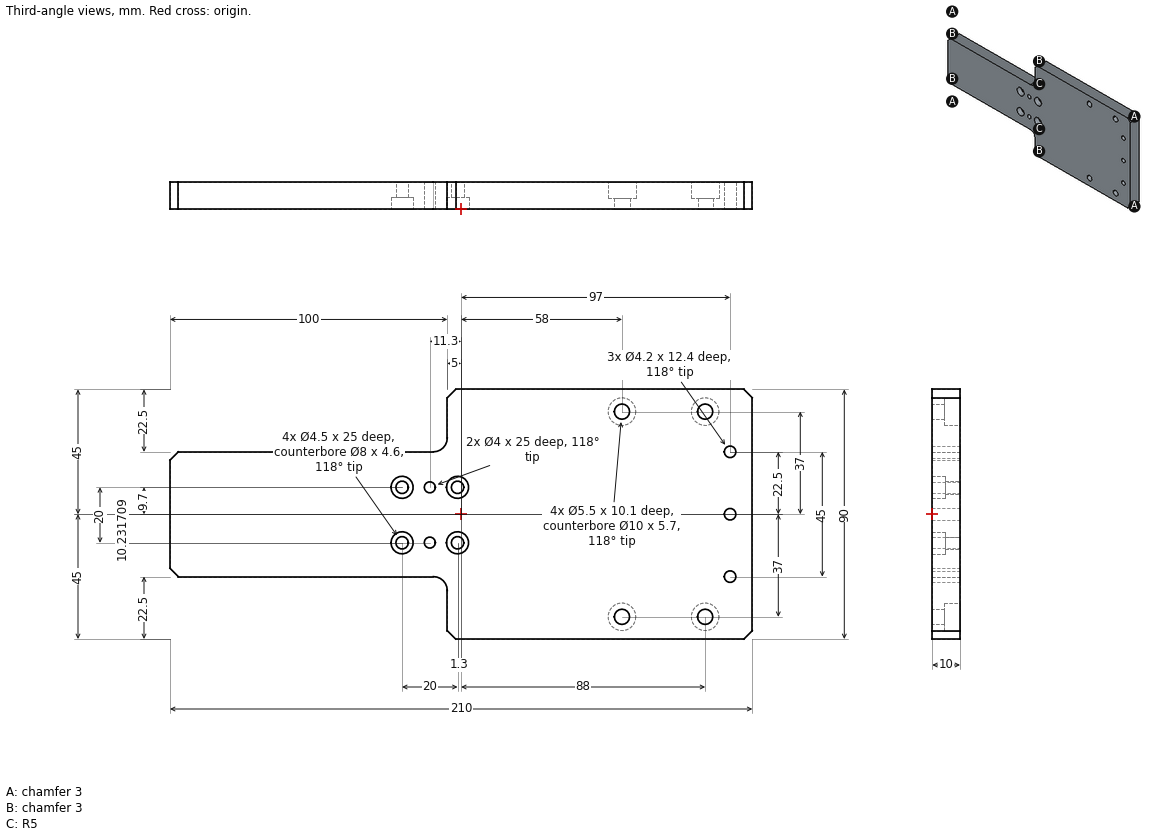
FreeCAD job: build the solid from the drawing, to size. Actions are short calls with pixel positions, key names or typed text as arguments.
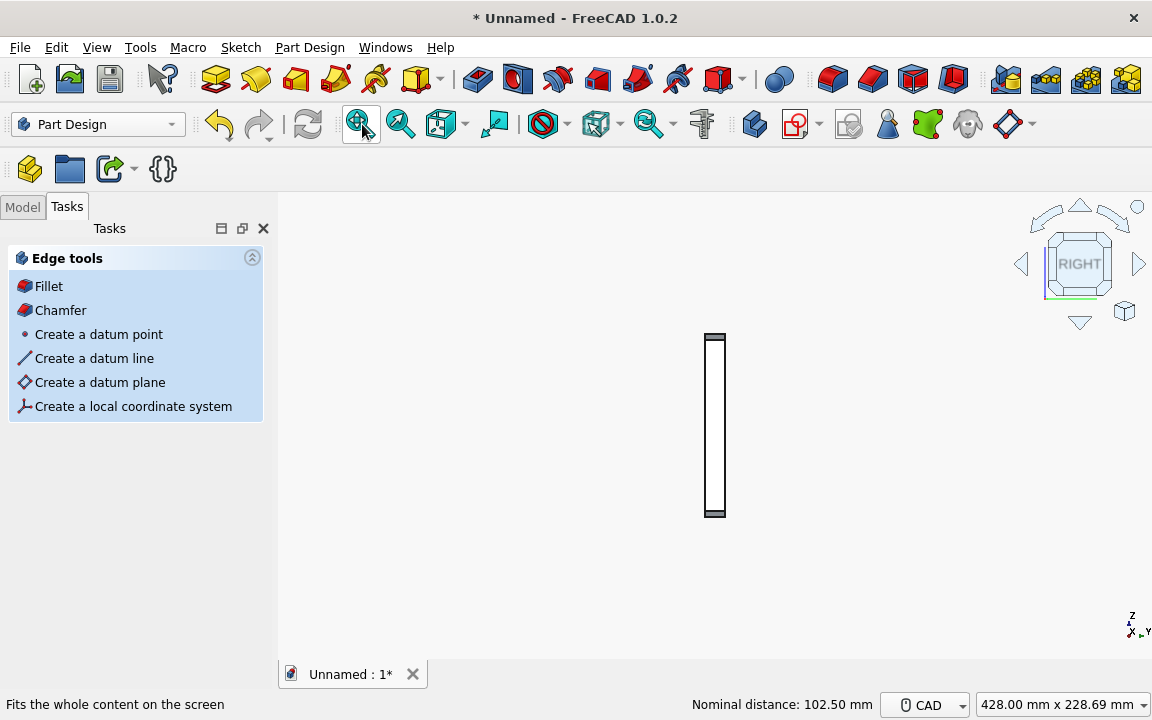
key(5)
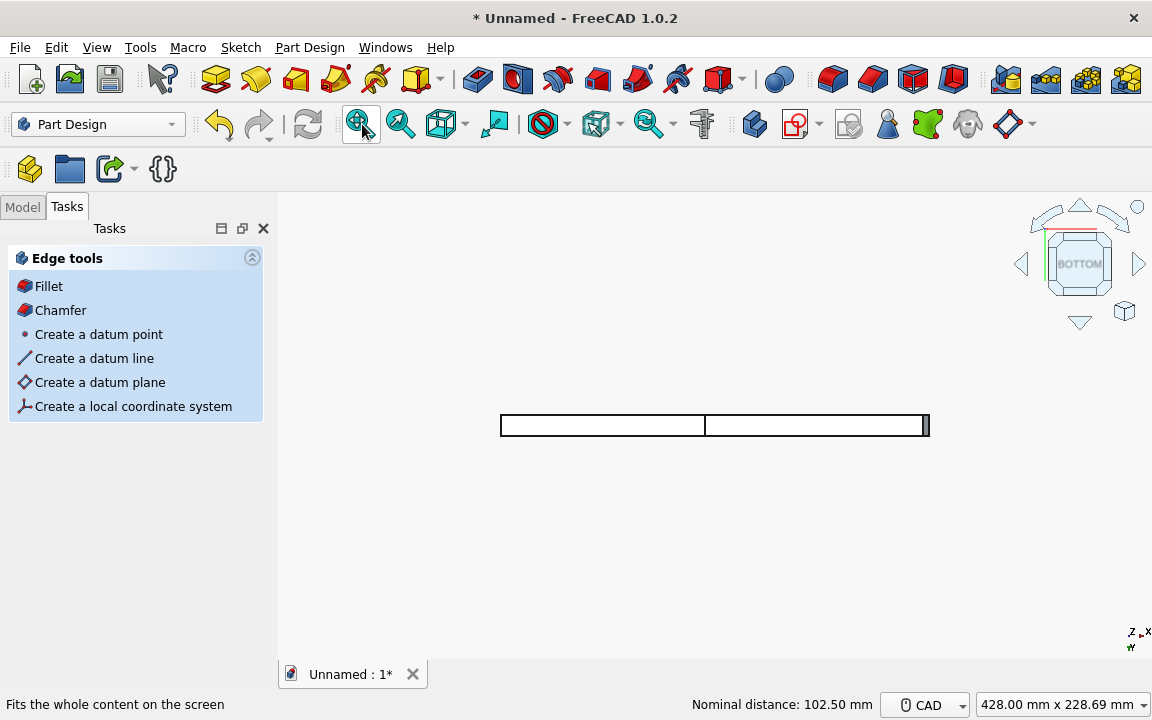
click(705, 424, ctrl)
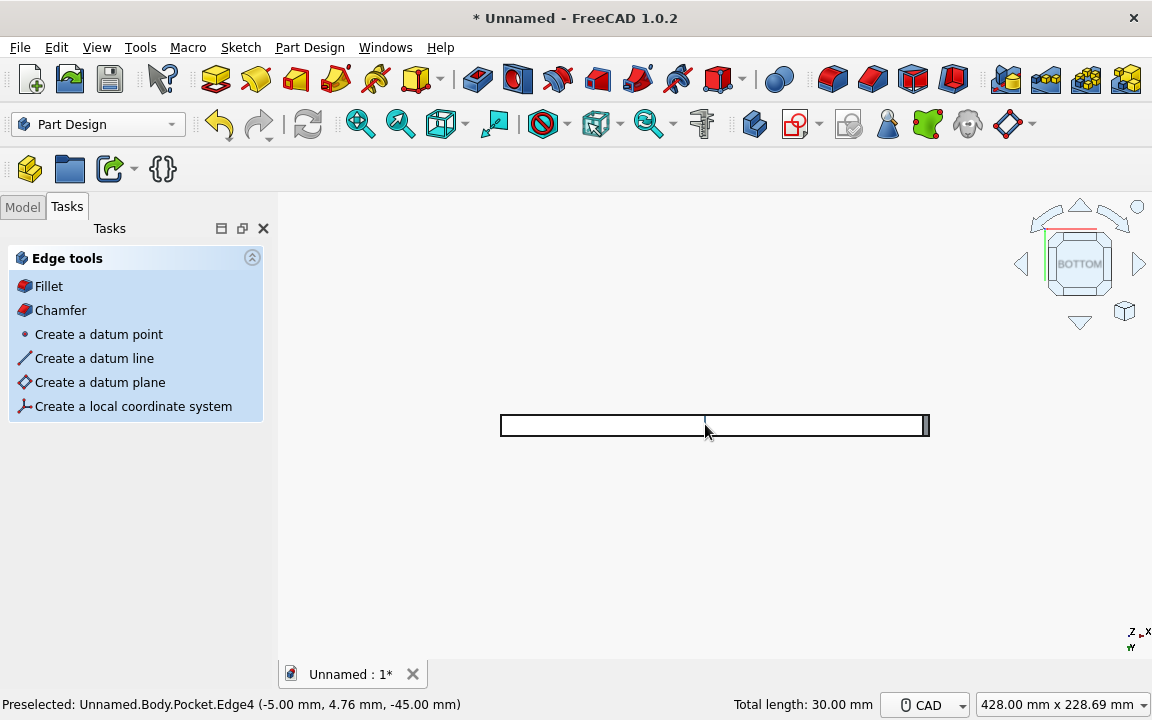
click(501, 424, ctrl)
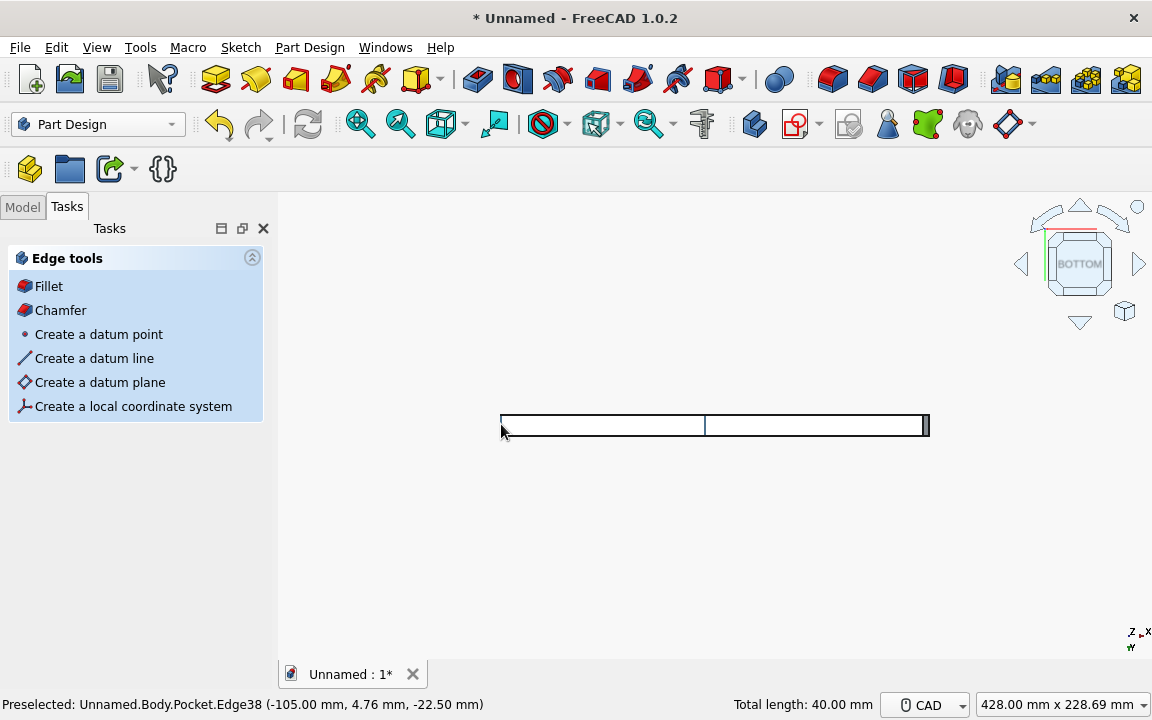
click(874, 80)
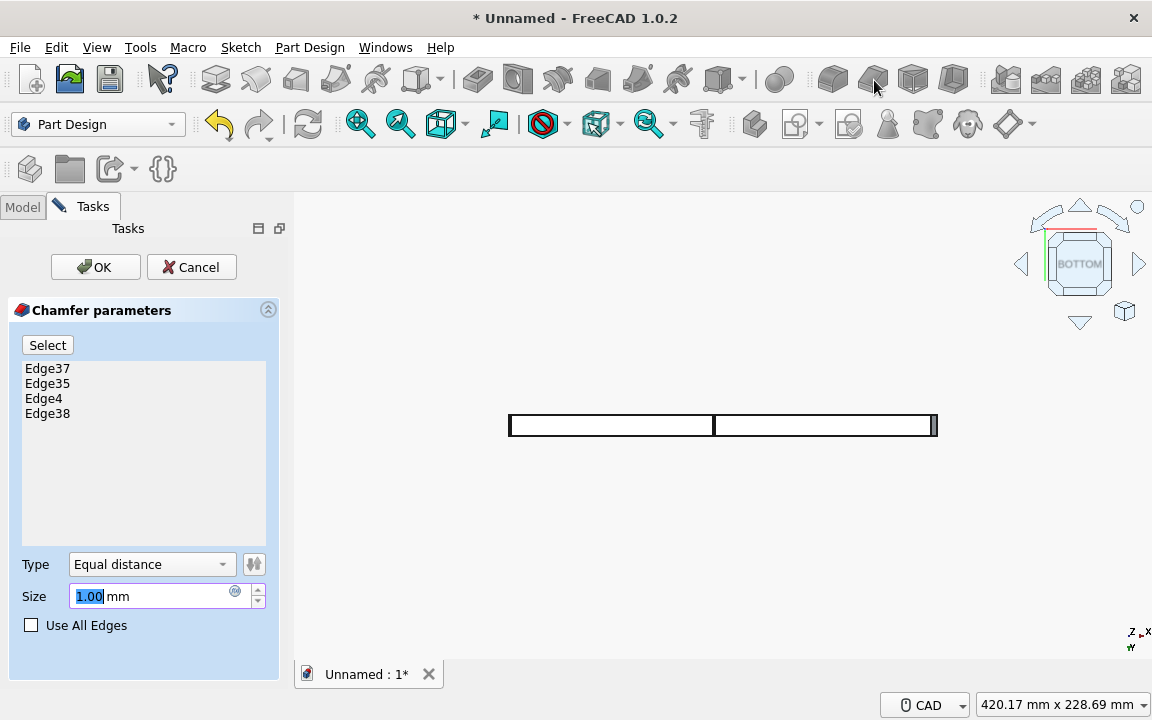
text(3)
key(Tab)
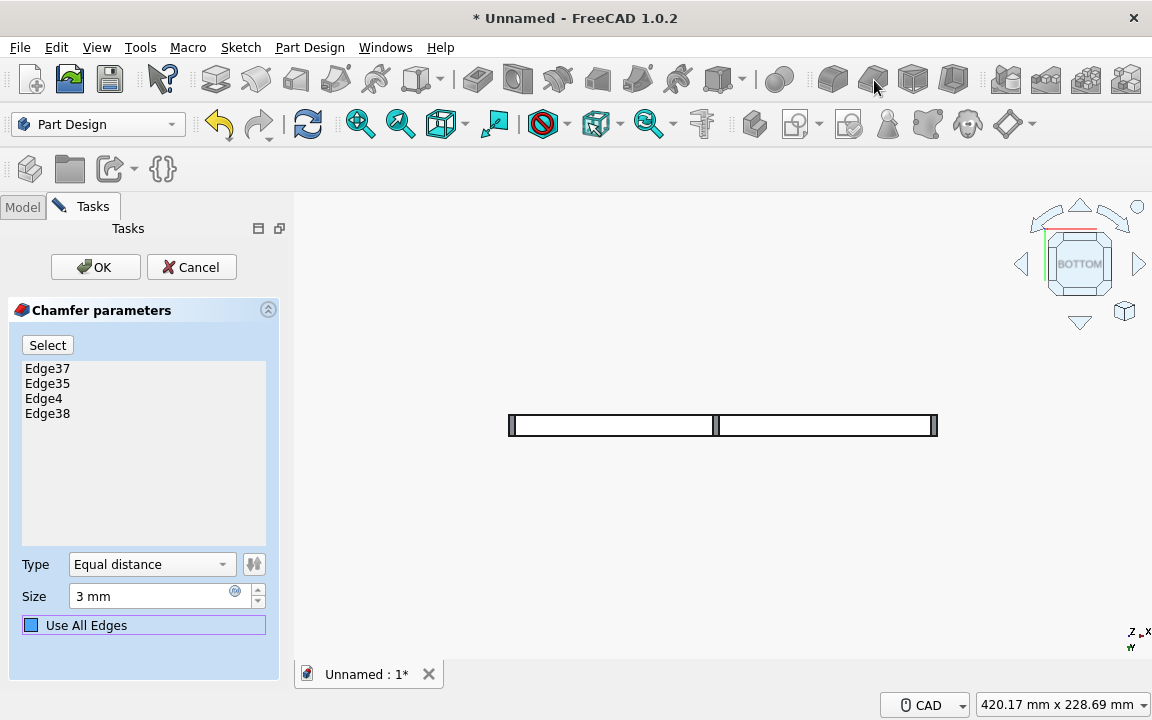
click(96, 267)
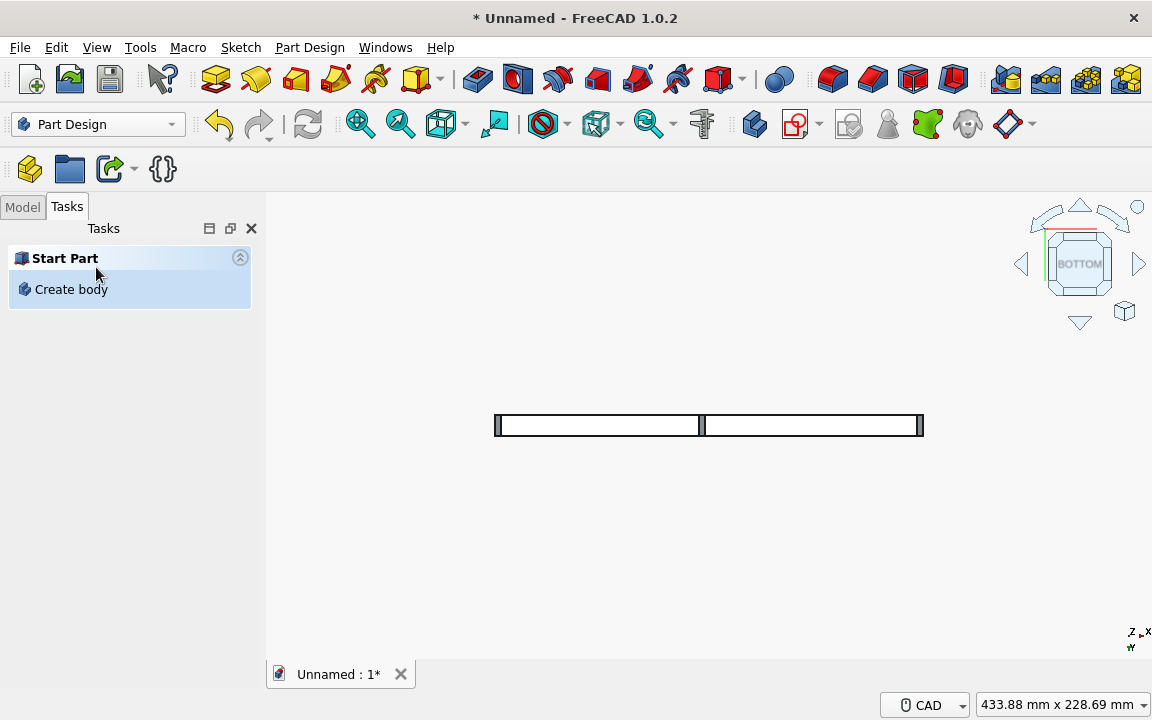
scroll(699, 424, up, 4)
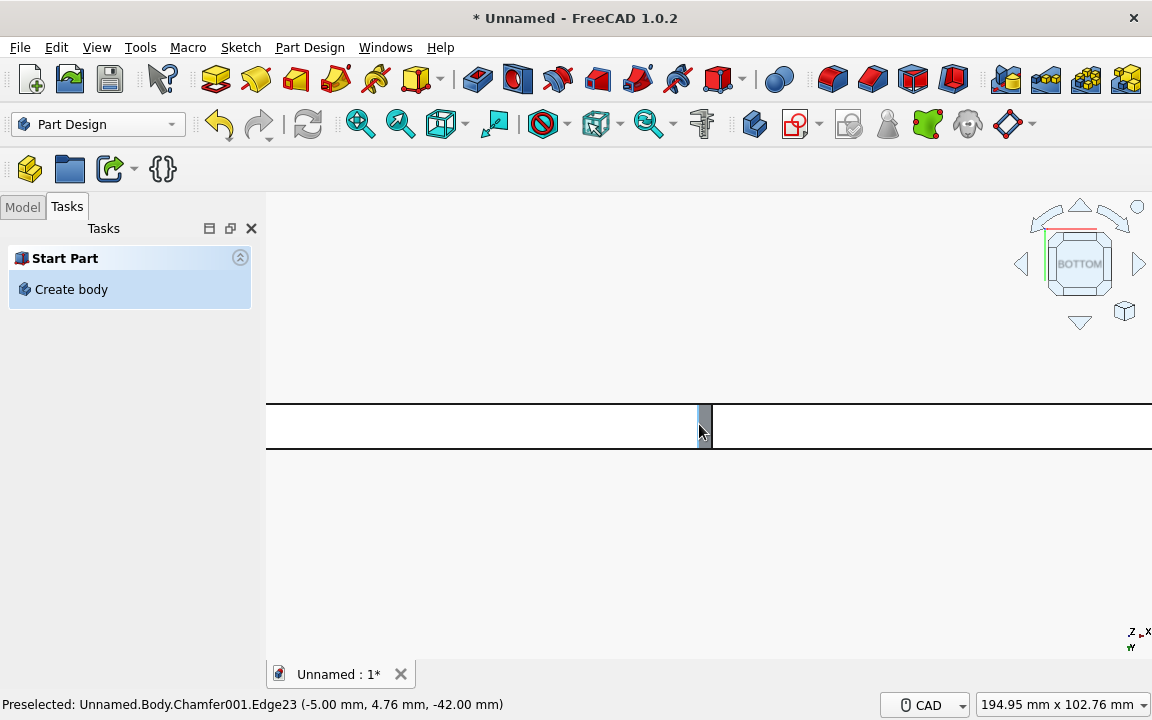
click(362, 124)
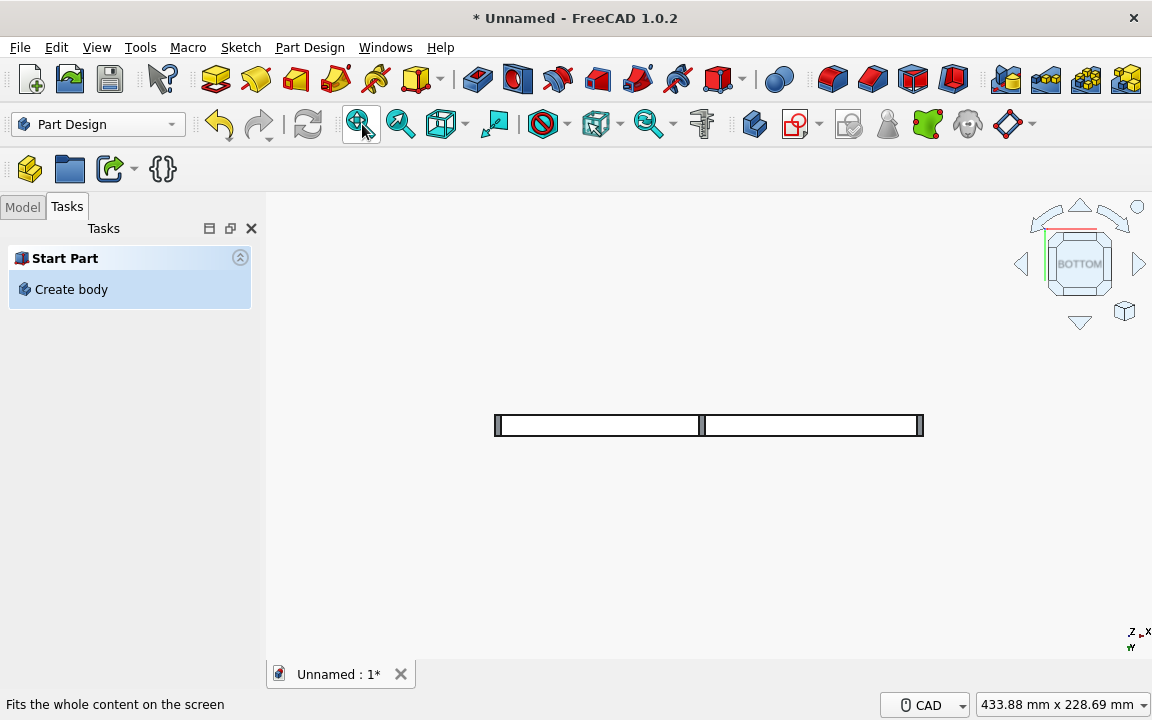
key(0)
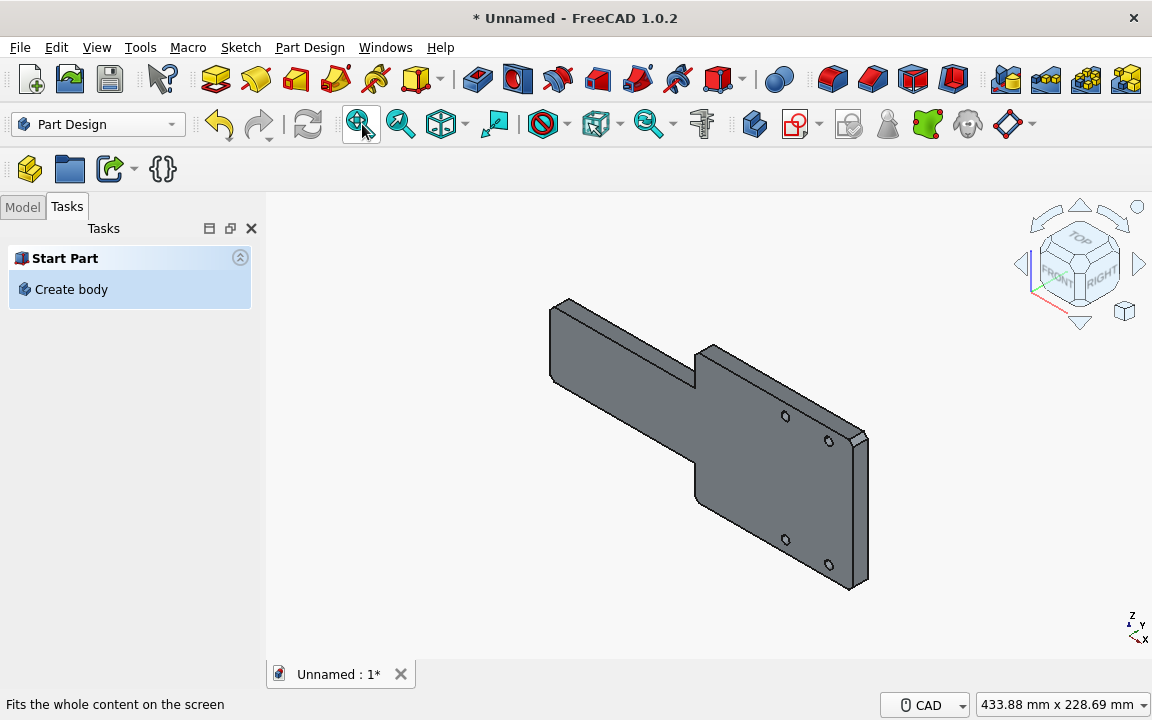
scroll(702, 383, up, 4)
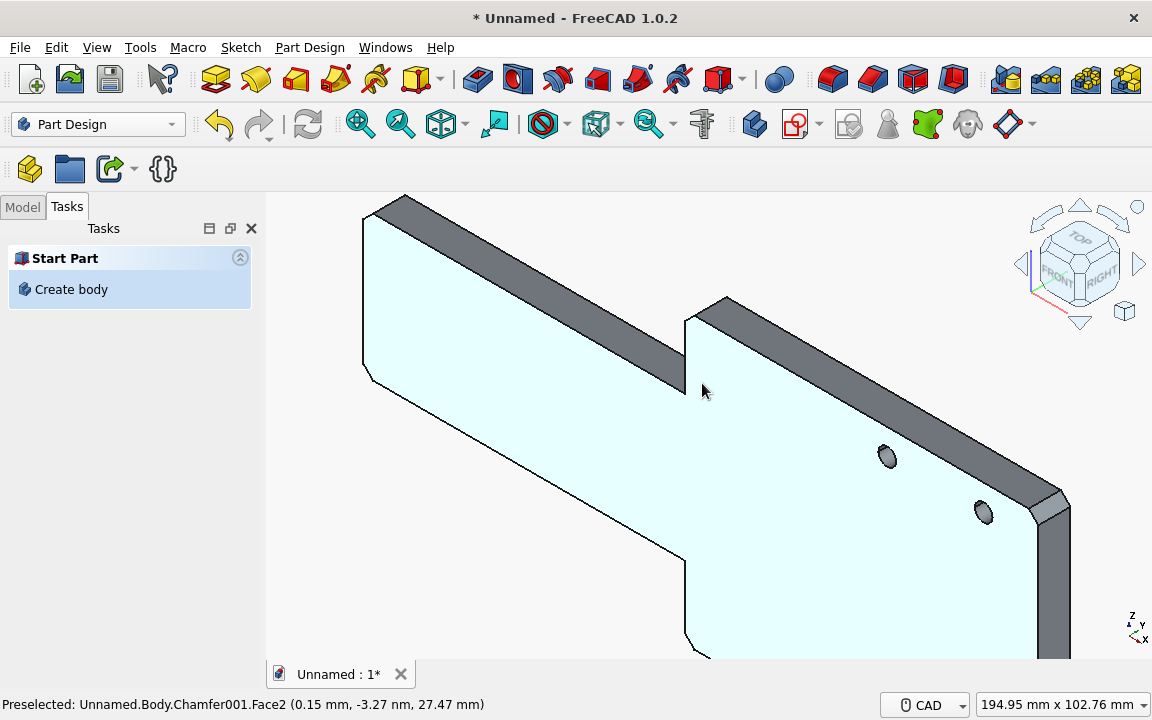
click(362, 124)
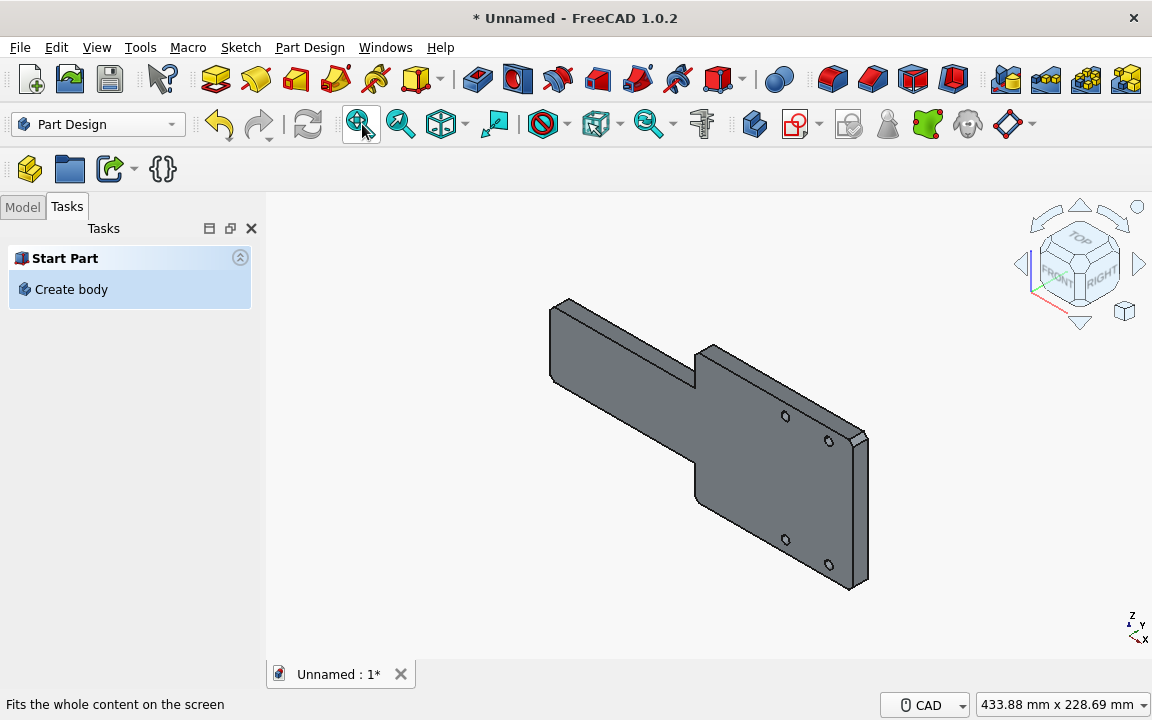
key(2)